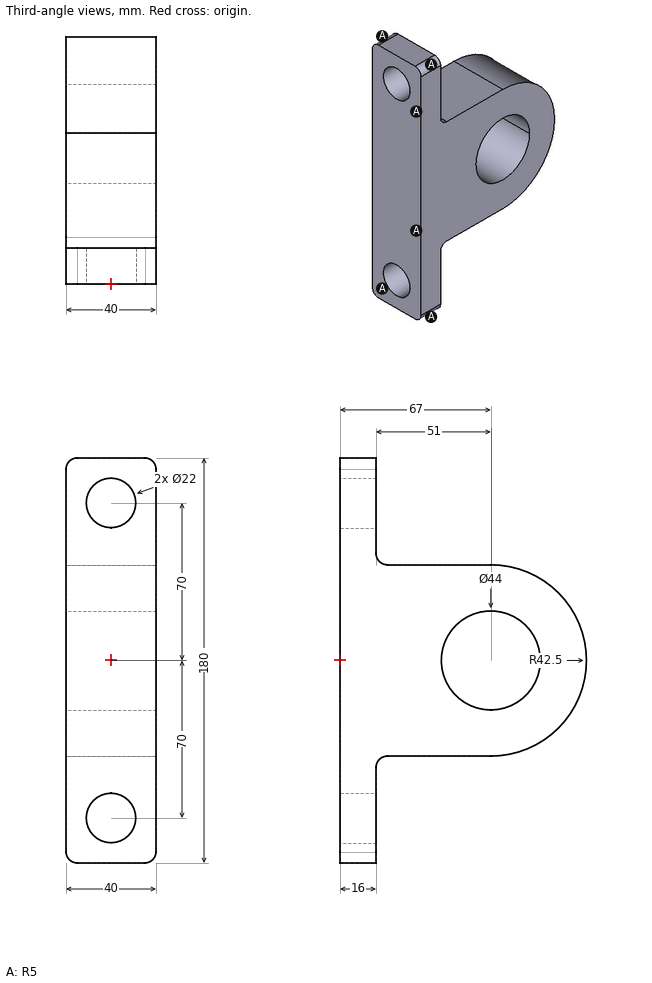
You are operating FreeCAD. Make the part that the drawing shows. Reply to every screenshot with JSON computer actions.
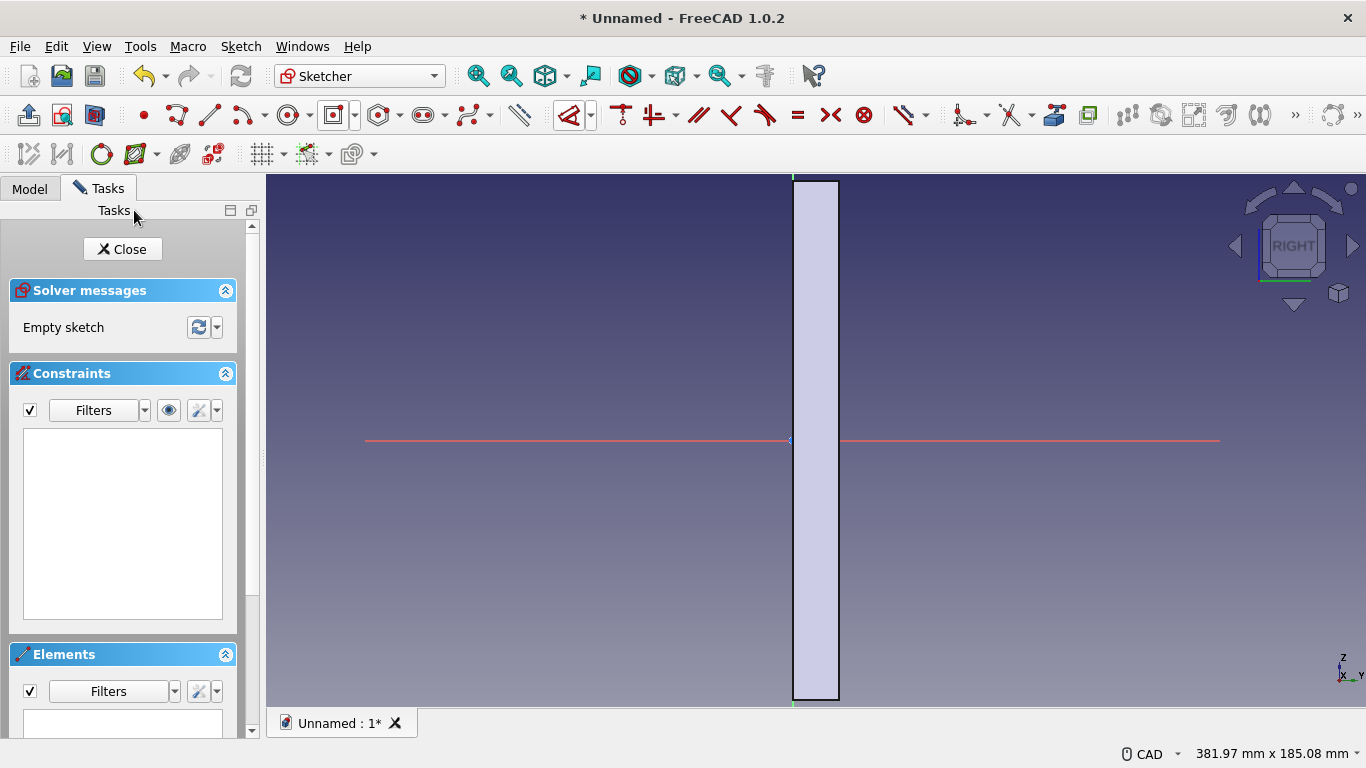
{"action": "left_click", "coordinate": [95, 116]}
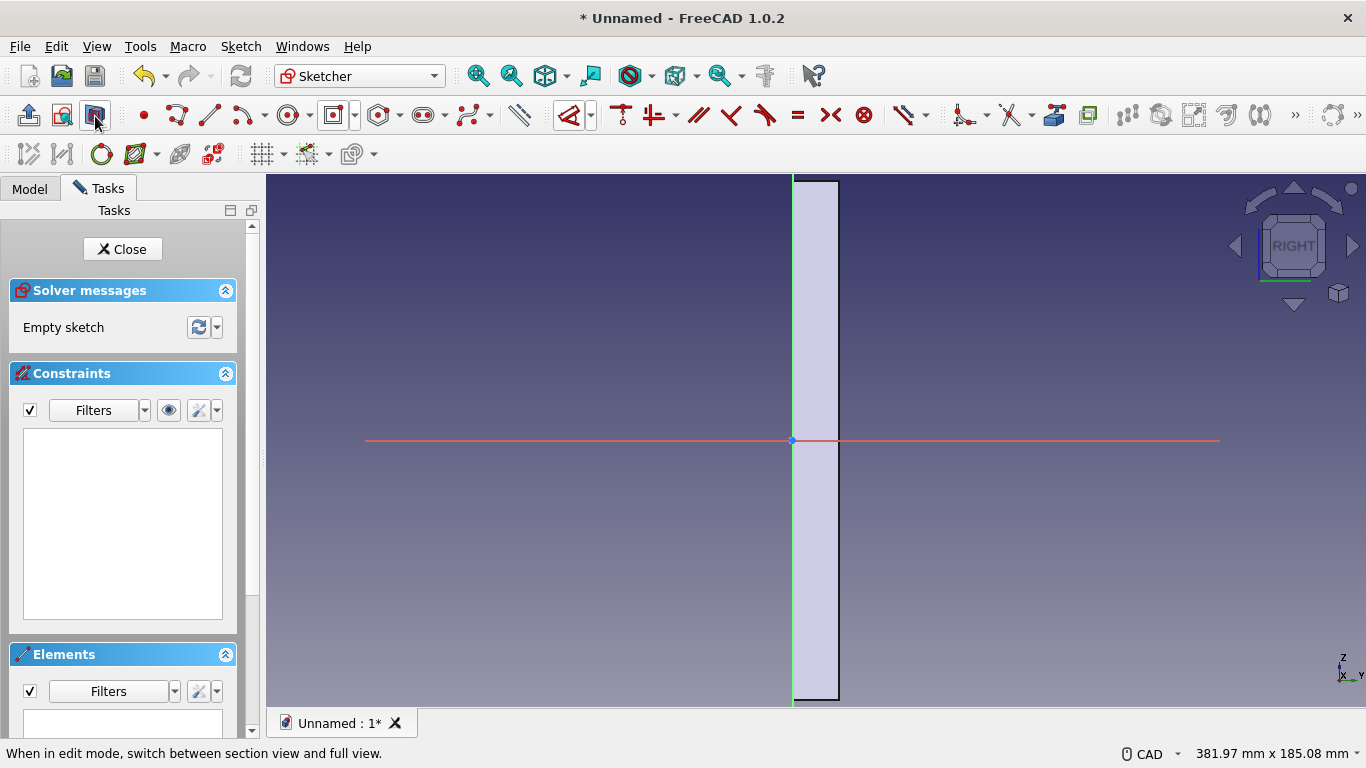
{"action": "scroll", "coordinate": [1201, 440], "scroll_direction": "up", "scroll_amount": 2}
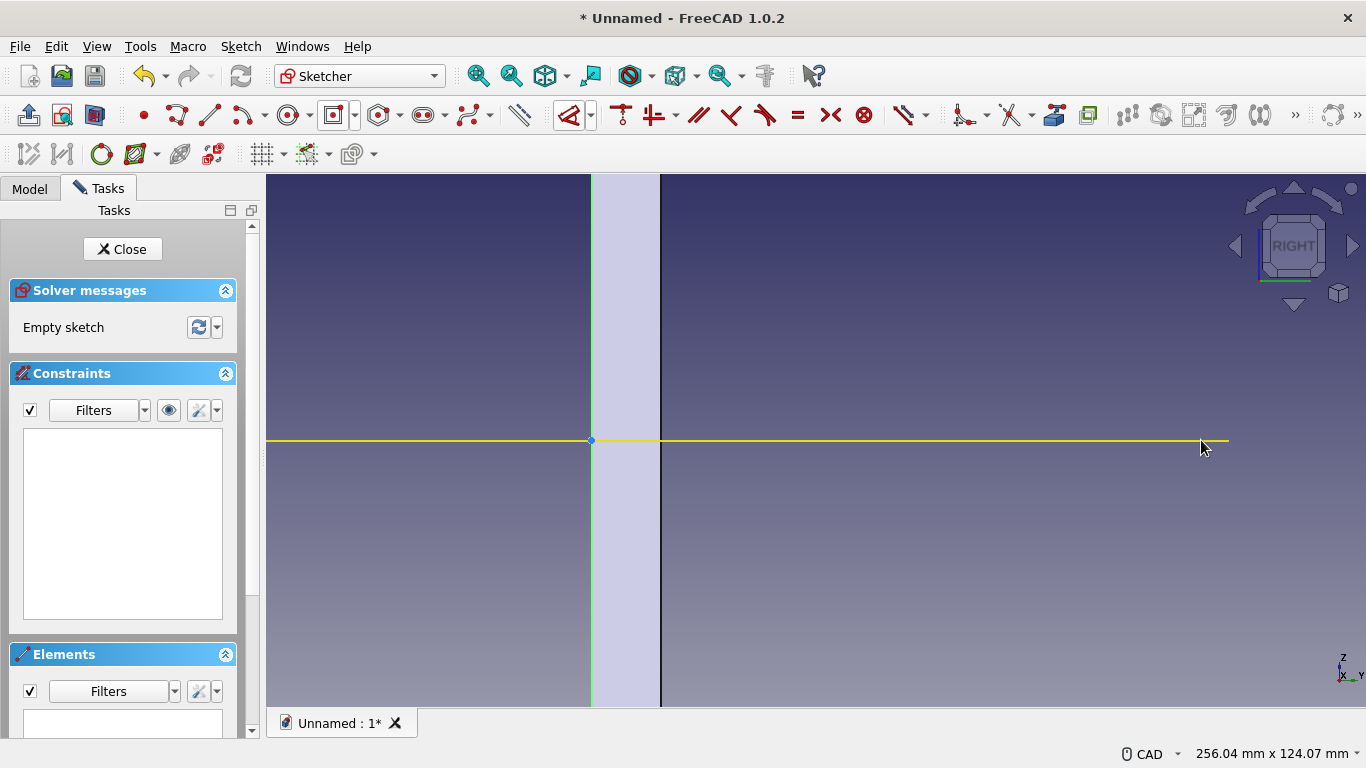
{"action": "left_click", "coordinate": [177, 116]}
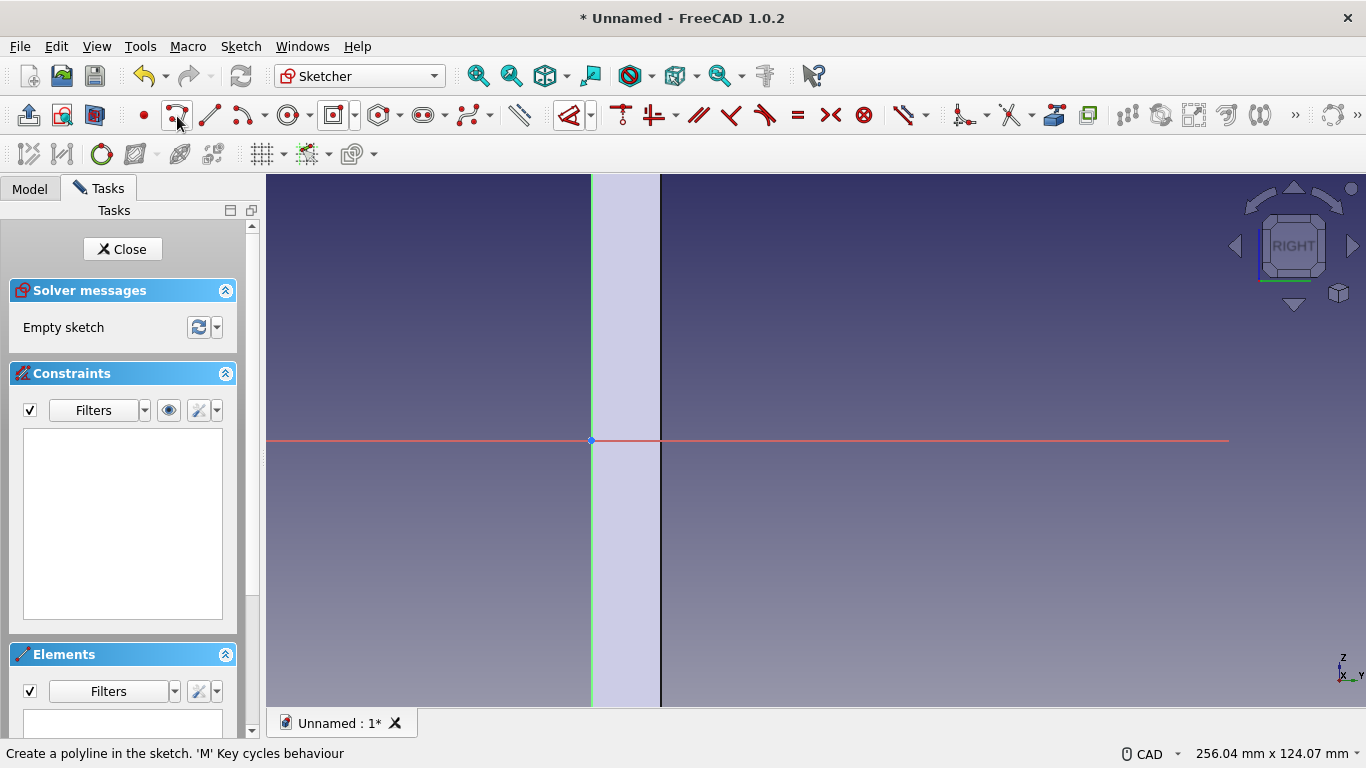
{"action": "left_click", "coordinate": [880, 258]}
{"action": "left_click", "coordinate": [661, 258]}
{"action": "left_click", "coordinate": [661, 623]}
{"action": "left_click", "coordinate": [880, 623]}
{"action": "right_click", "coordinate": [880, 623]}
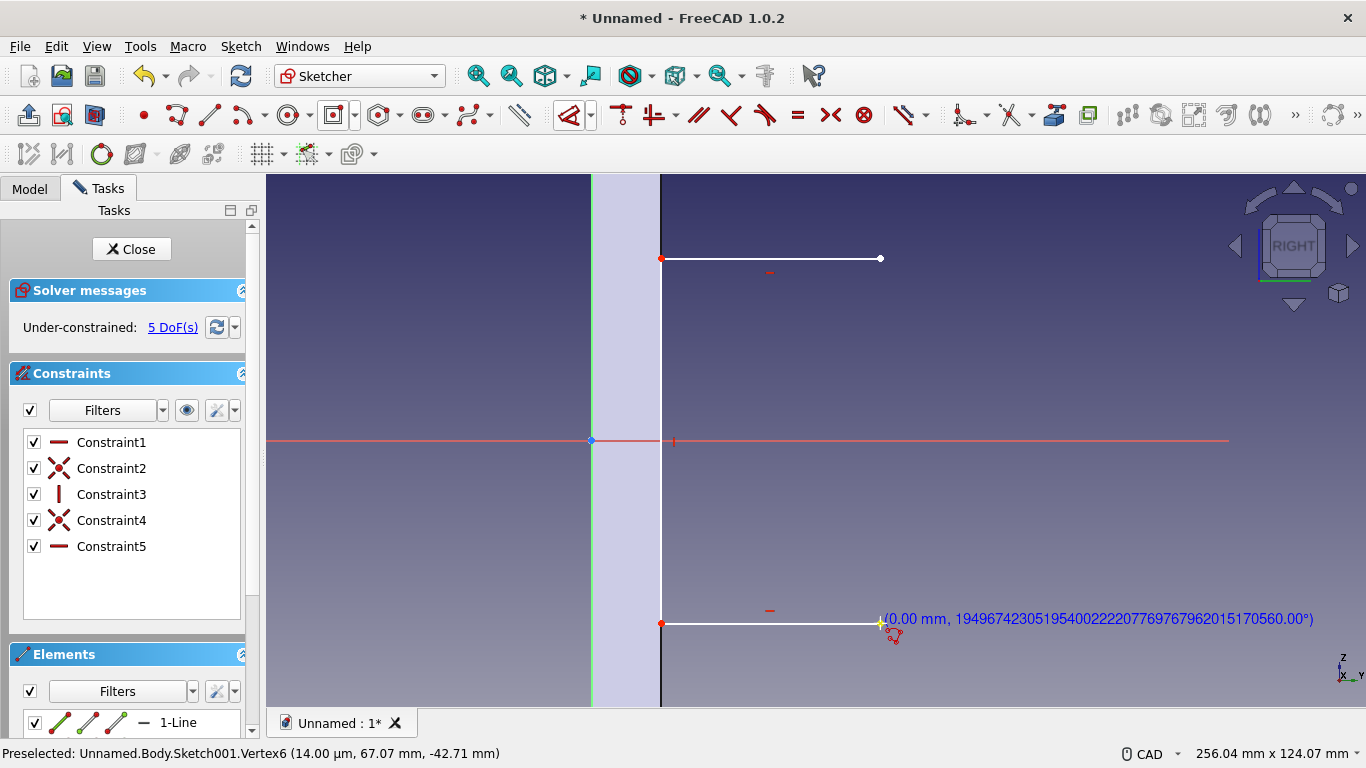
{"action": "key", "text": "g 3 a"}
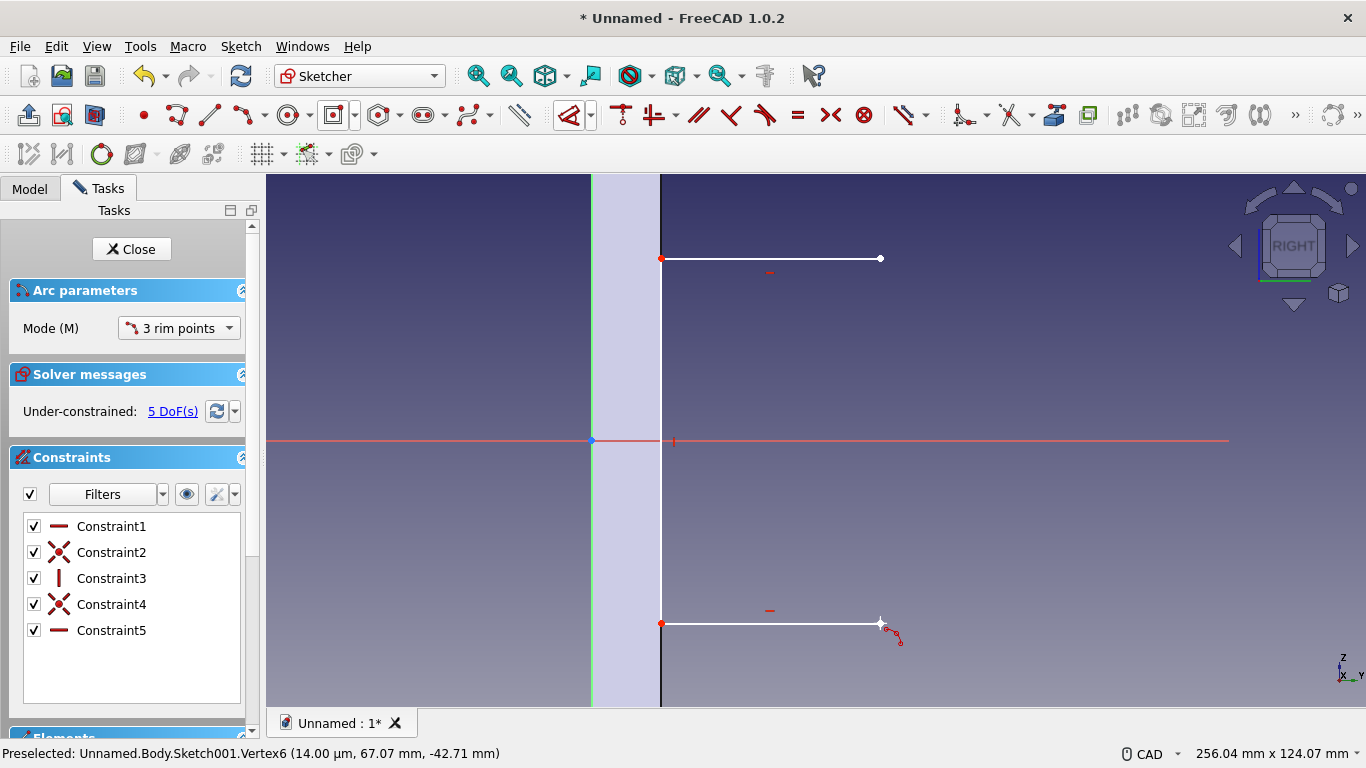
{"action": "left_click", "coordinate": [880, 624]}
{"action": "left_click", "coordinate": [880, 259]}
{"action": "left_click", "coordinate": [1053, 497]}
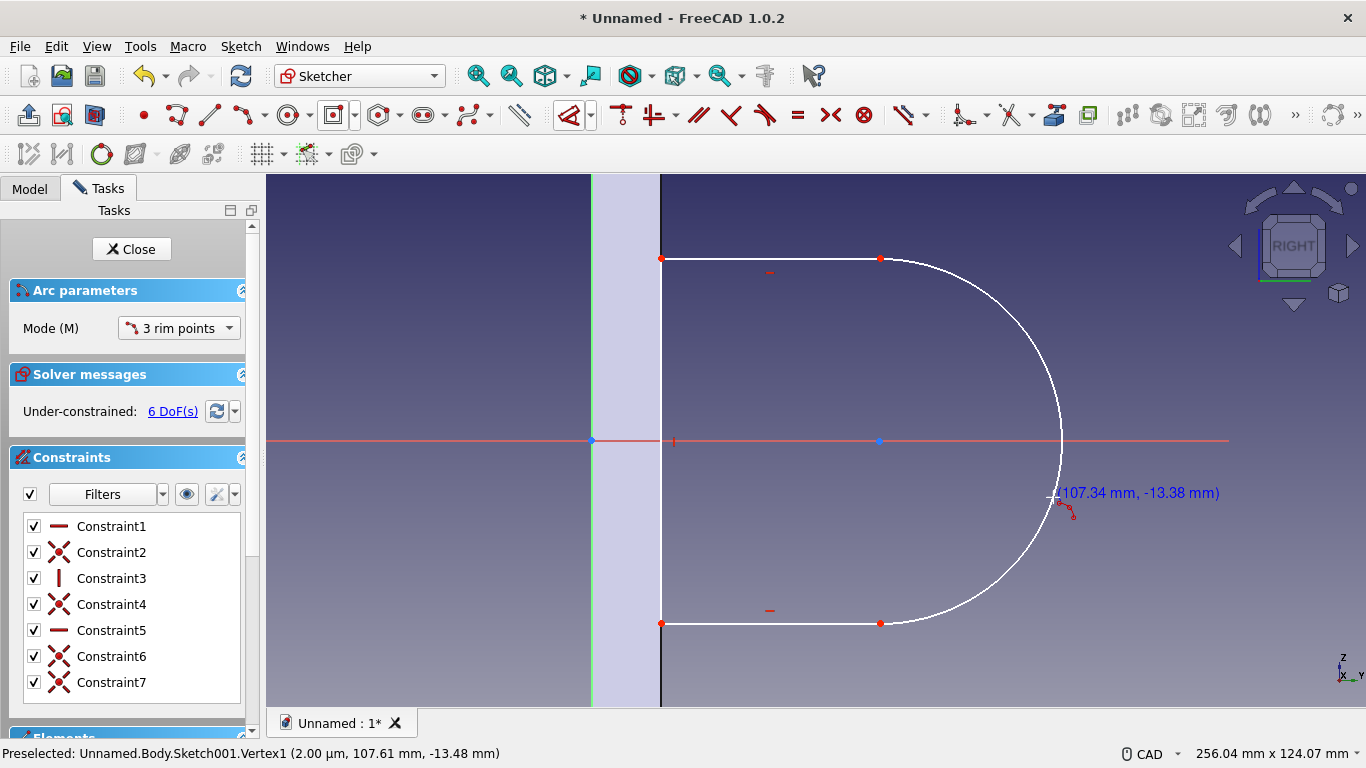
{"action": "key", "text": "g c"}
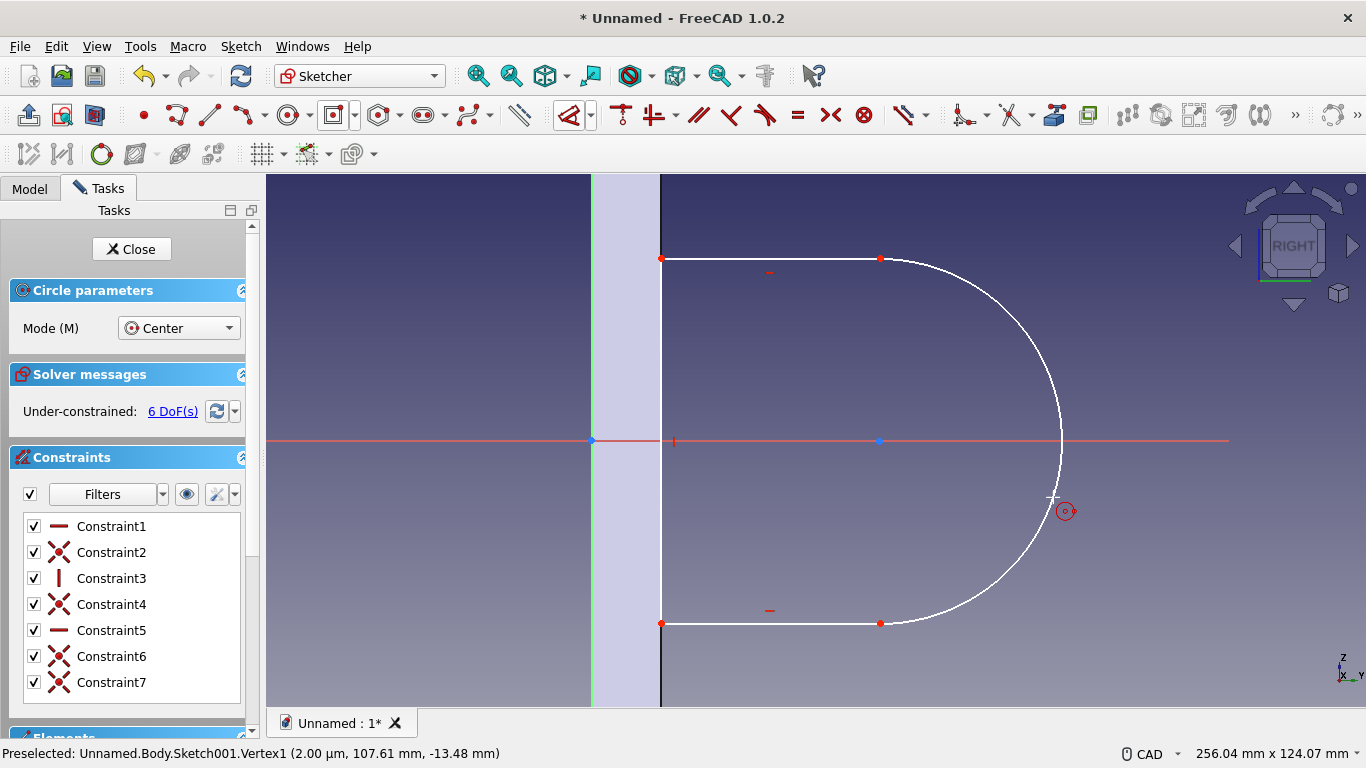
{"action": "left_click", "coordinate": [880, 440]}
{"action": "mouse_move", "coordinate": [947, 374]}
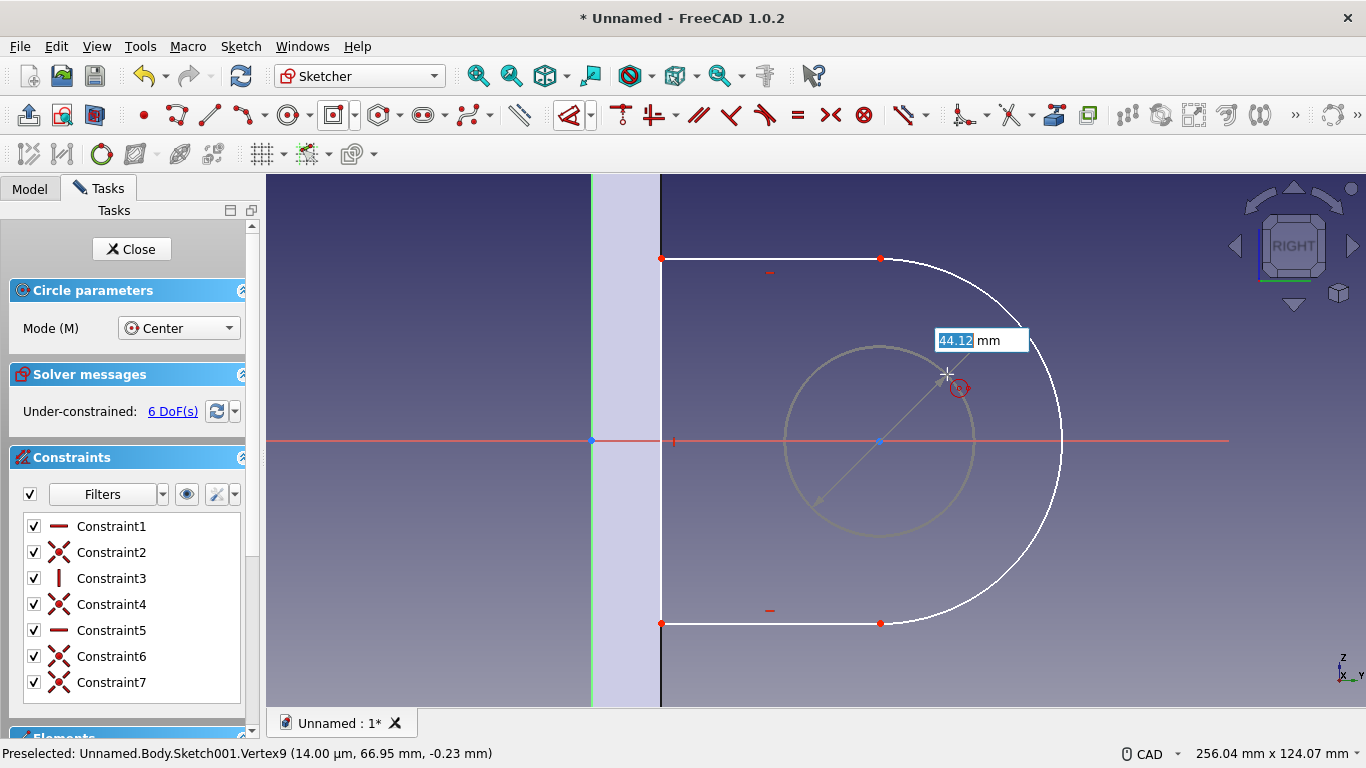
{"action": "type", "text": "44"}
{"action": "key", "text": "Return"}
{"action": "key", "text": "Escape"}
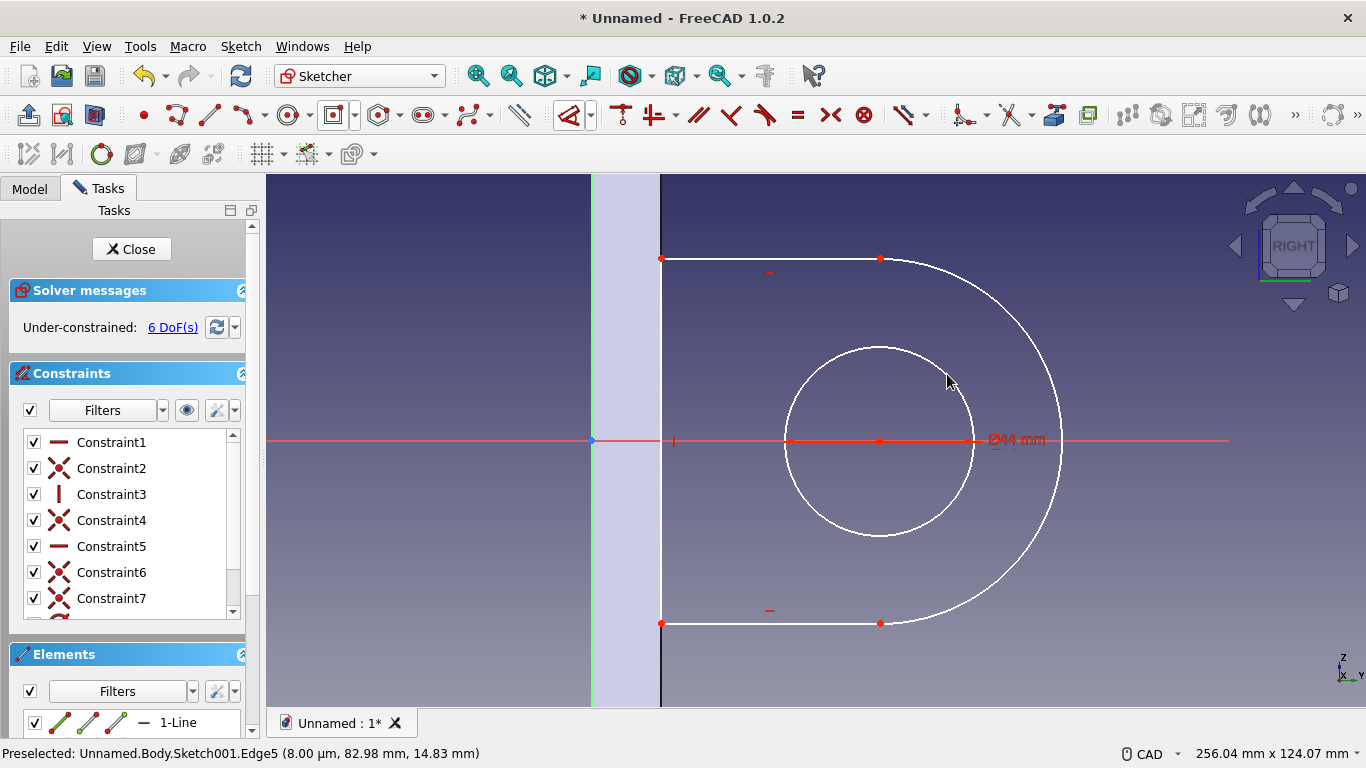
{"action": "left_click", "coordinate": [879, 442]}